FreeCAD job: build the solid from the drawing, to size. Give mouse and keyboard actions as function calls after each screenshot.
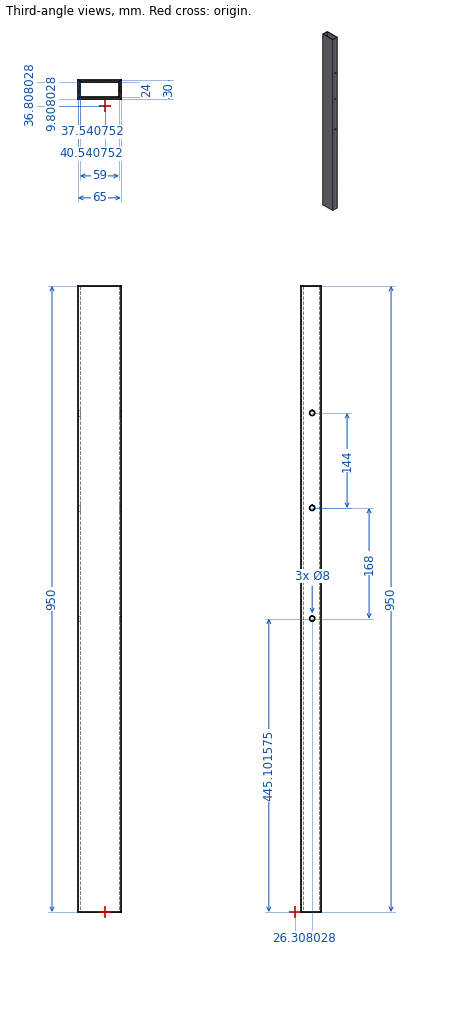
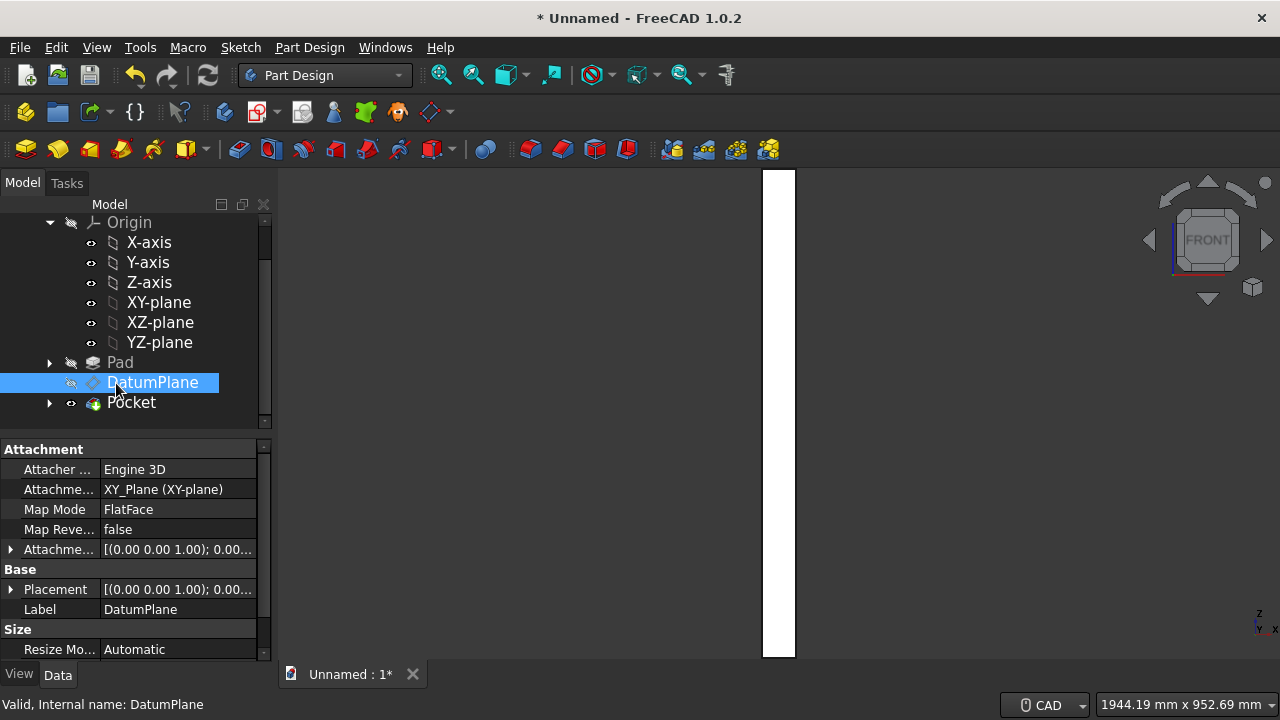
key(6)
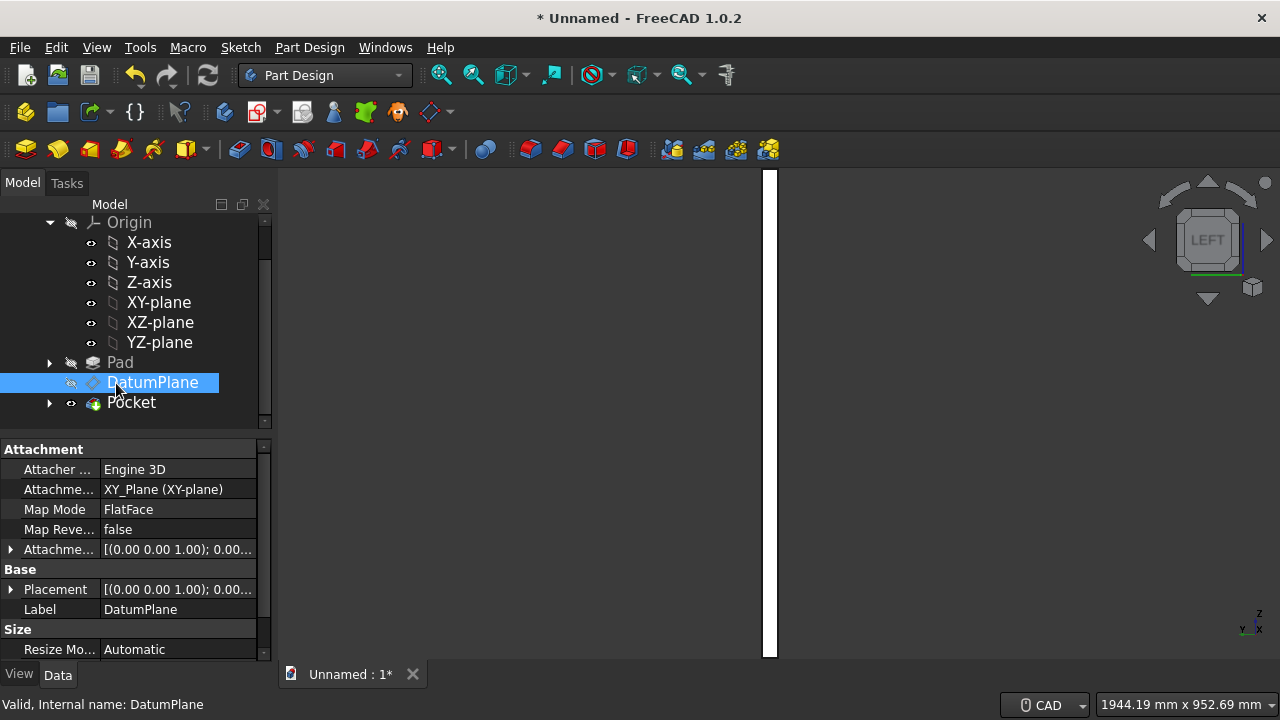
key(2)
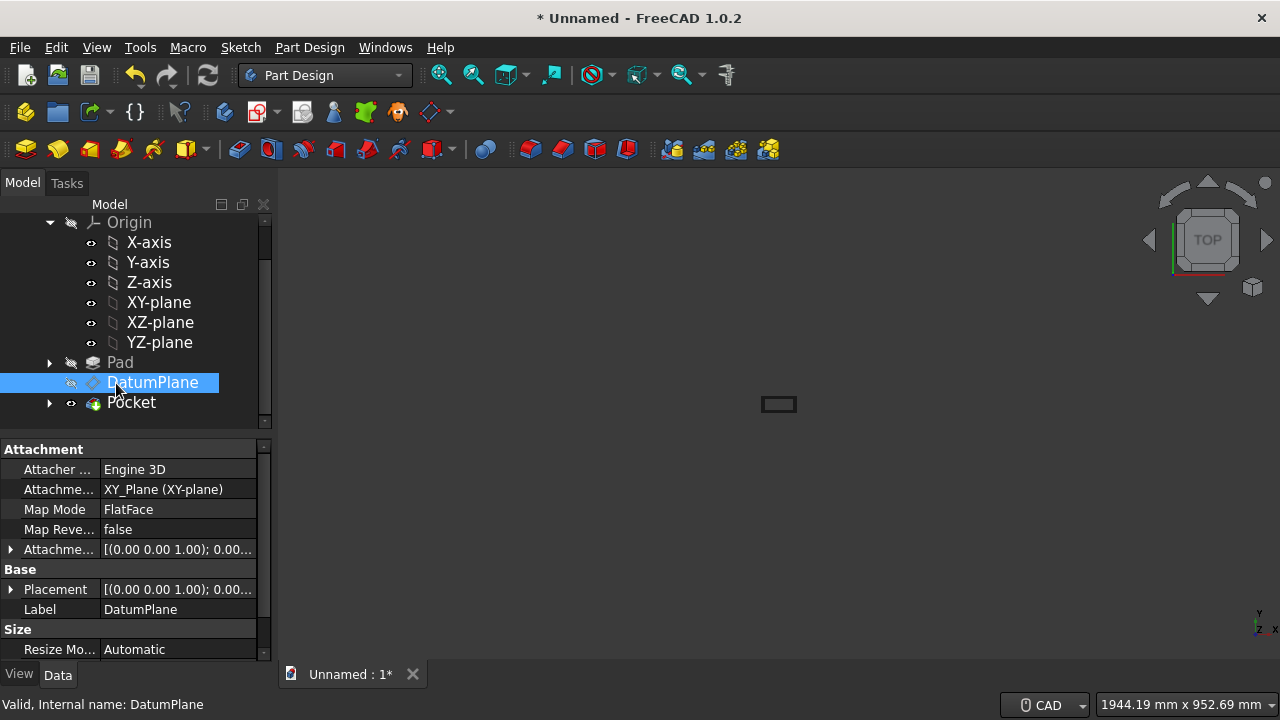
click(442, 76)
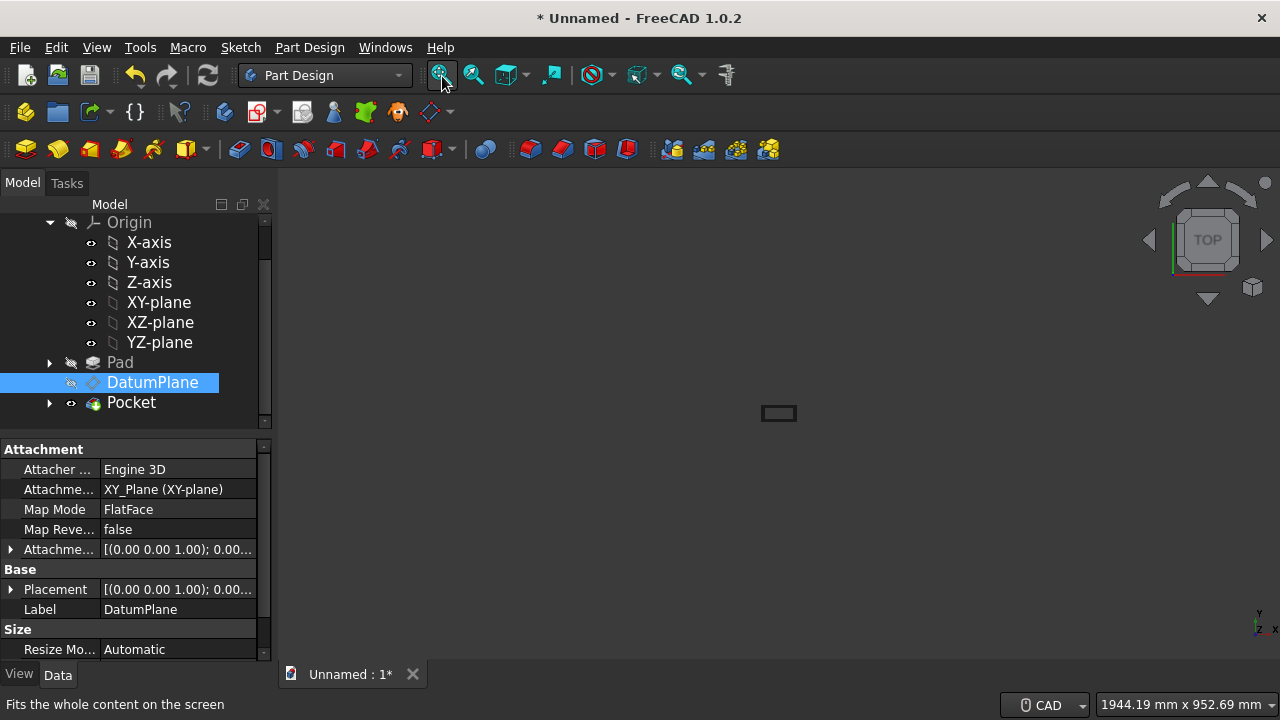
key(1)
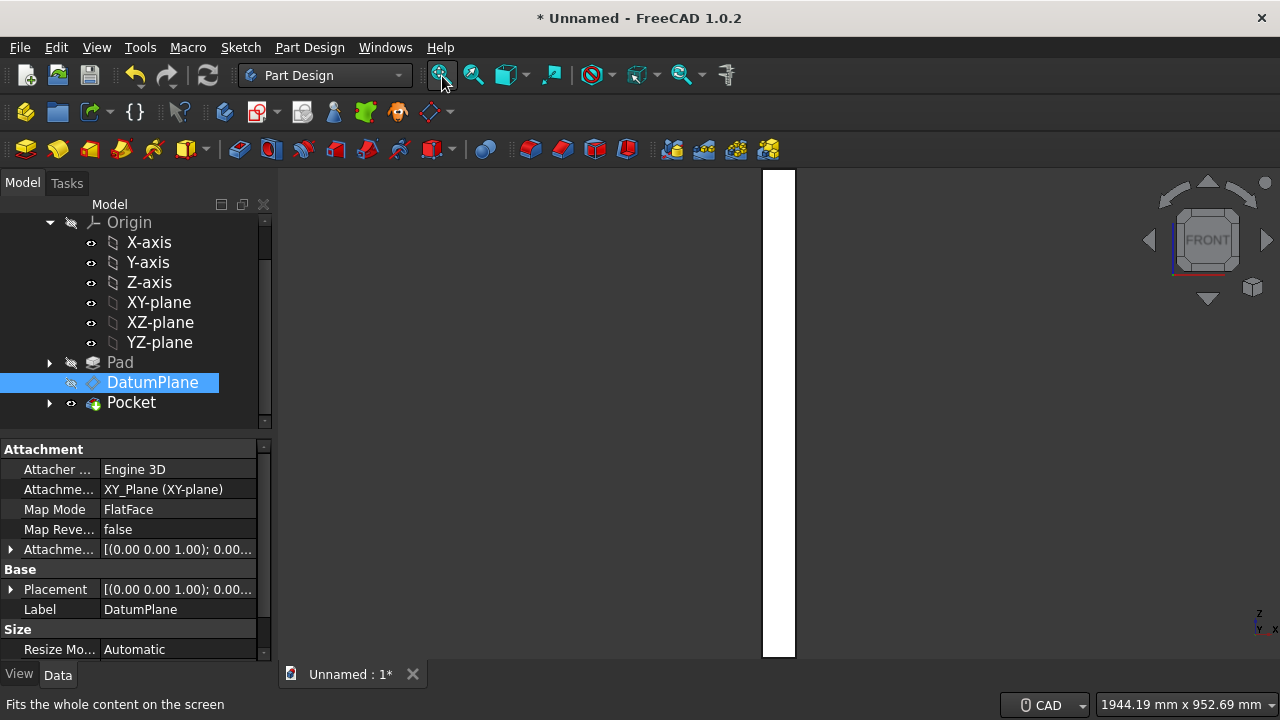
click(136, 343)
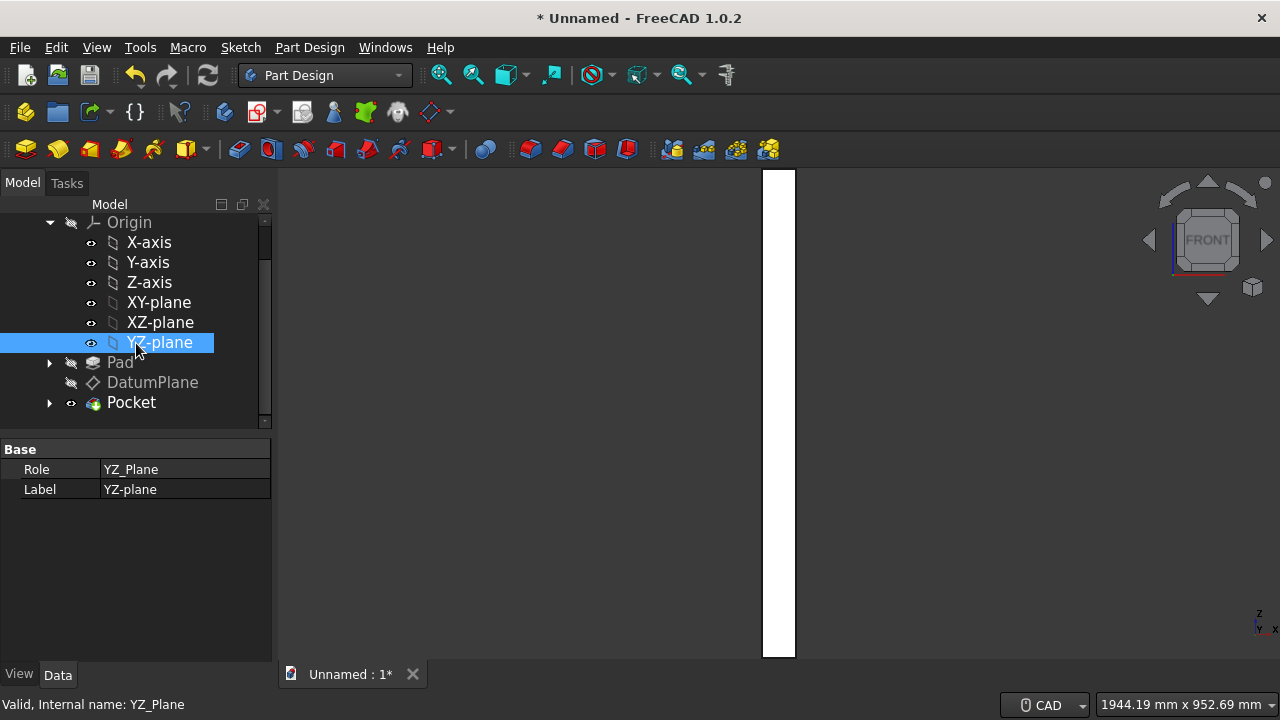
click(430, 112)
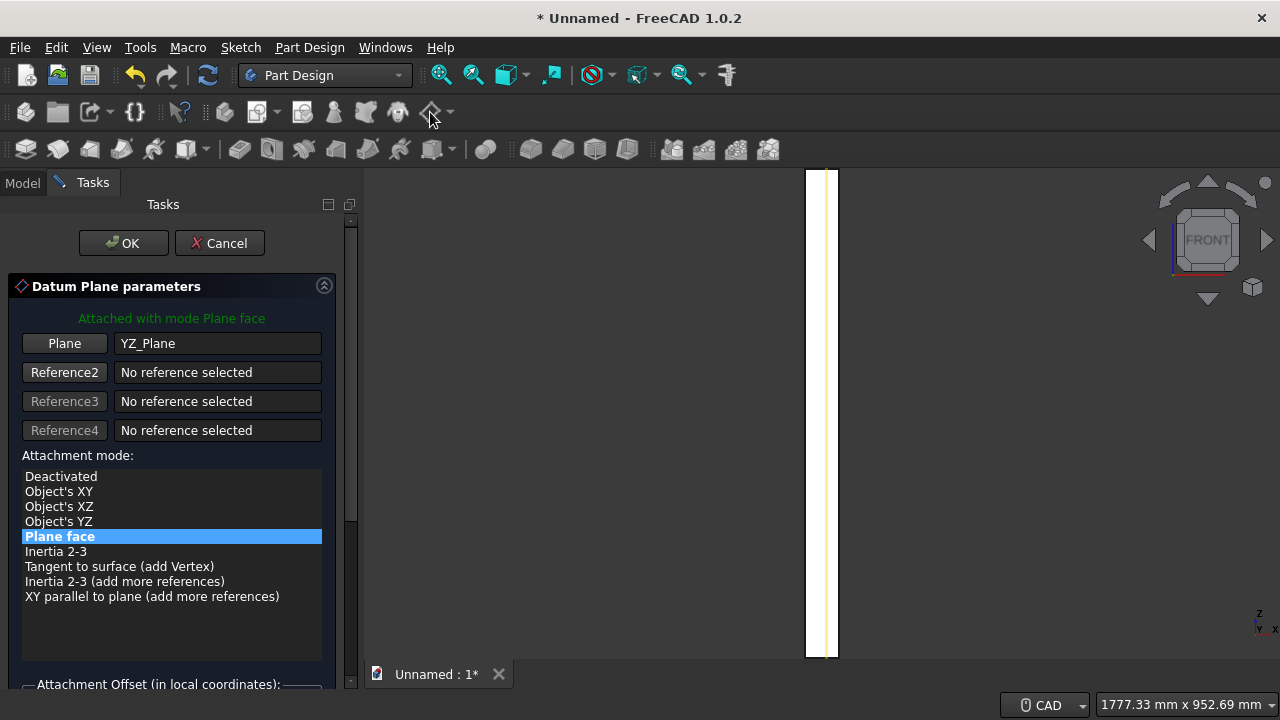
scroll(351, 451, down, 3)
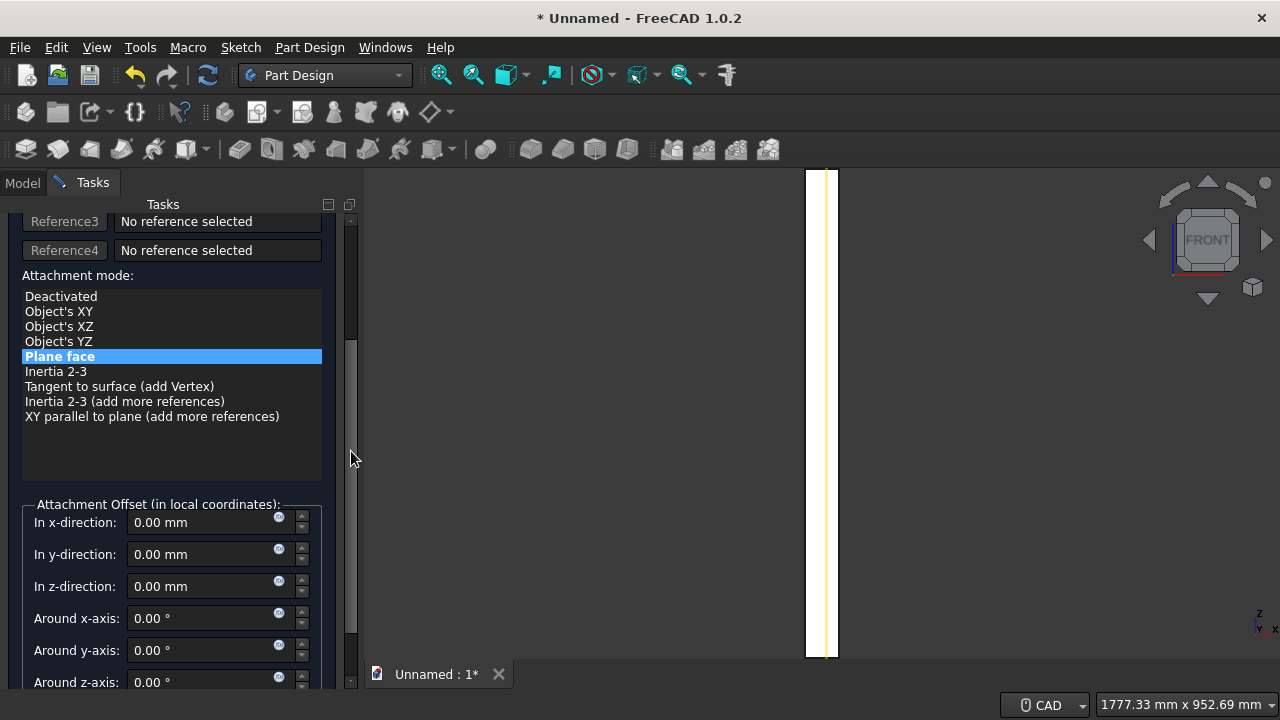
triple_click(210, 586)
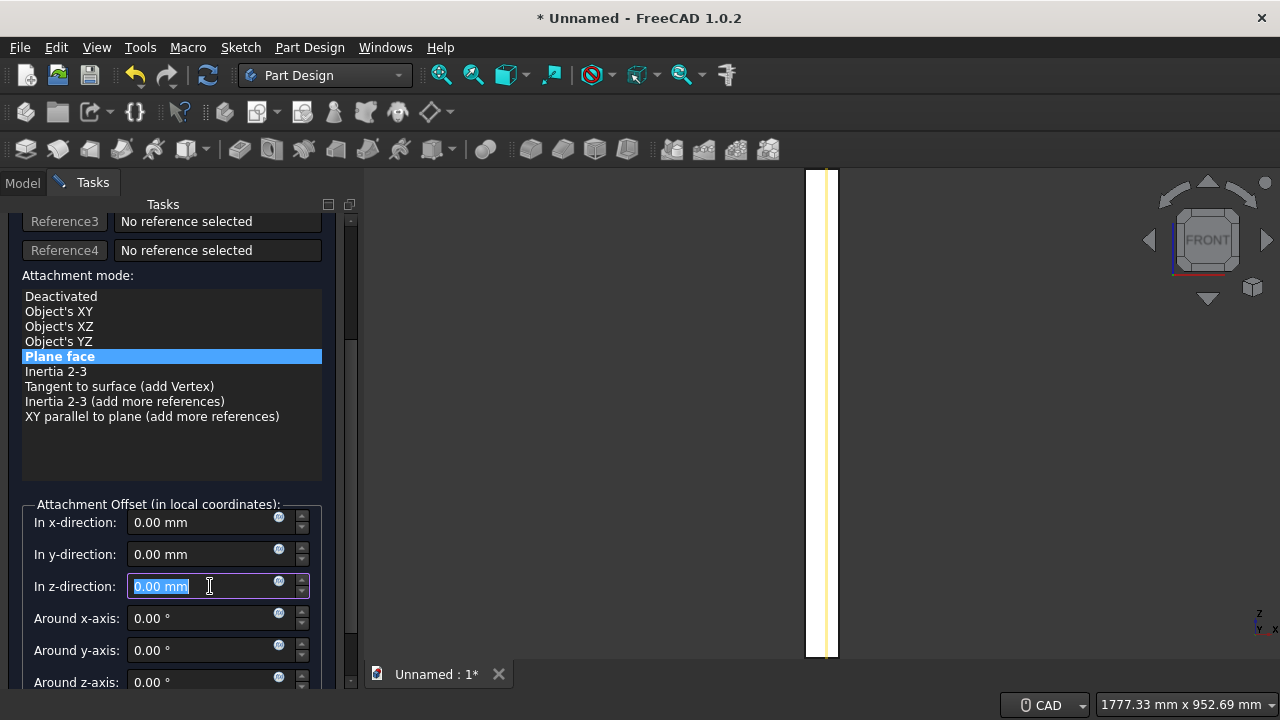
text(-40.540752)
key(Tab)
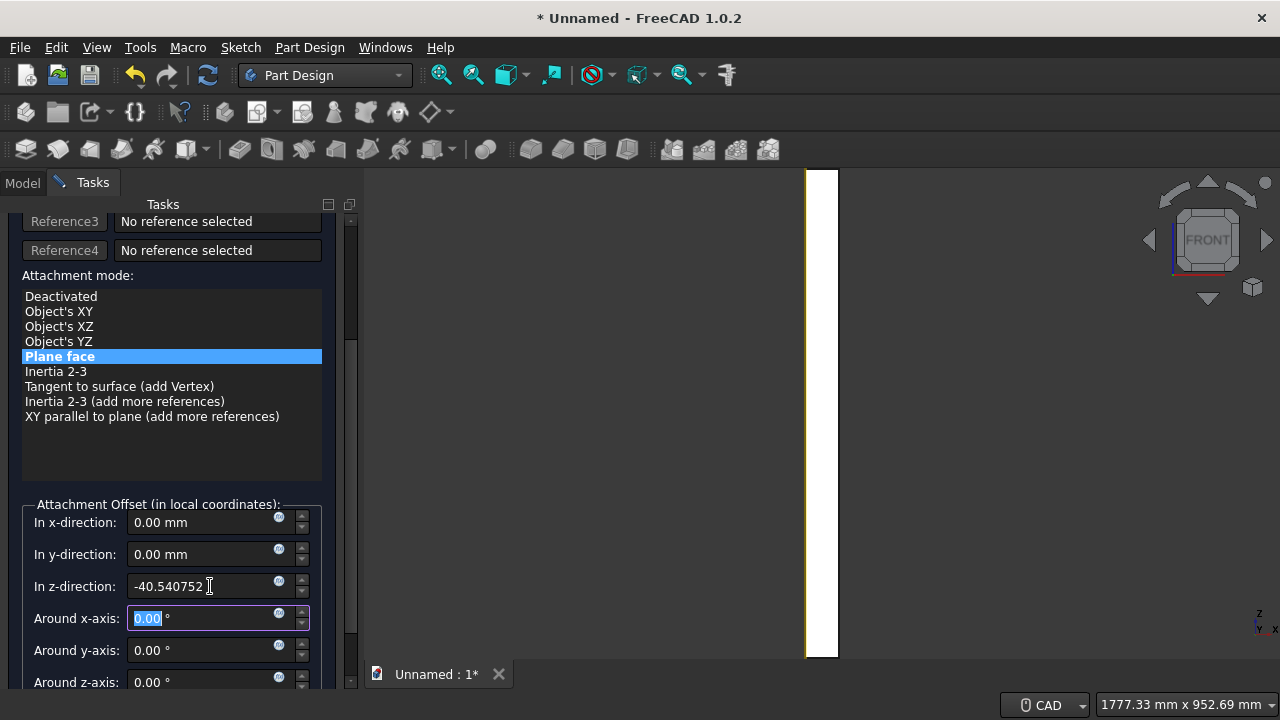
scroll(351, 451, up, 4)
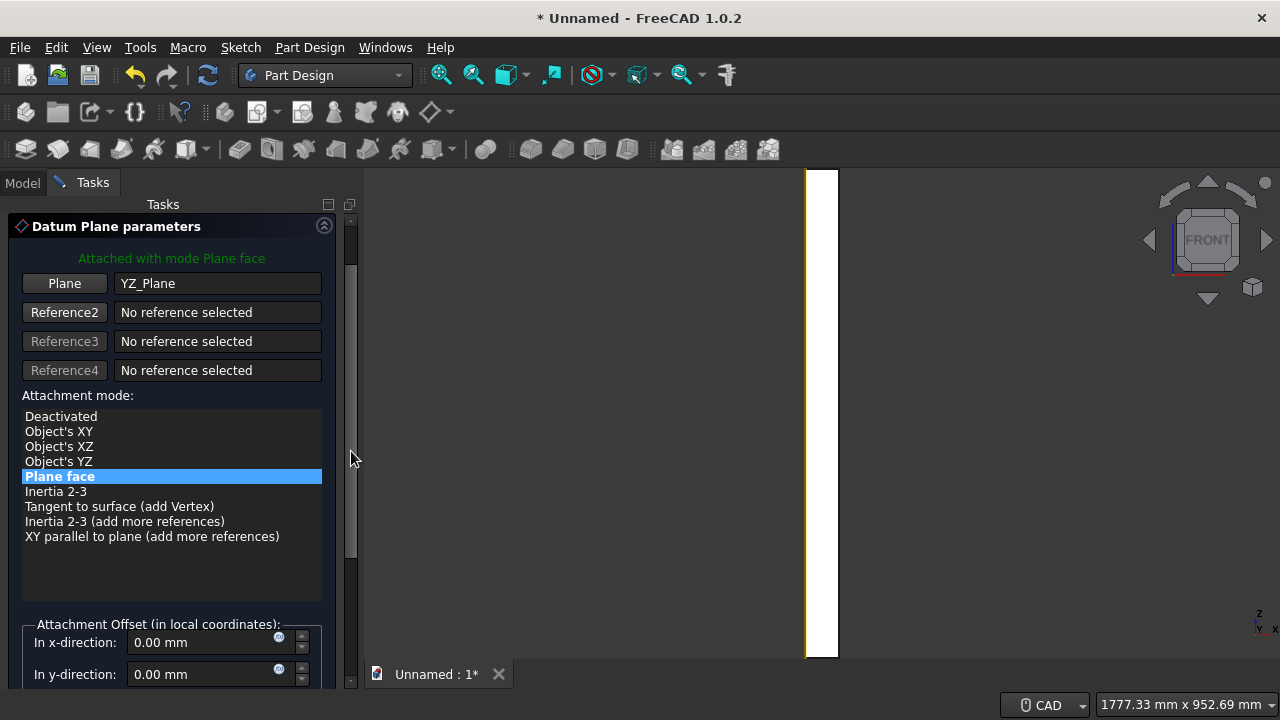
click(124, 243)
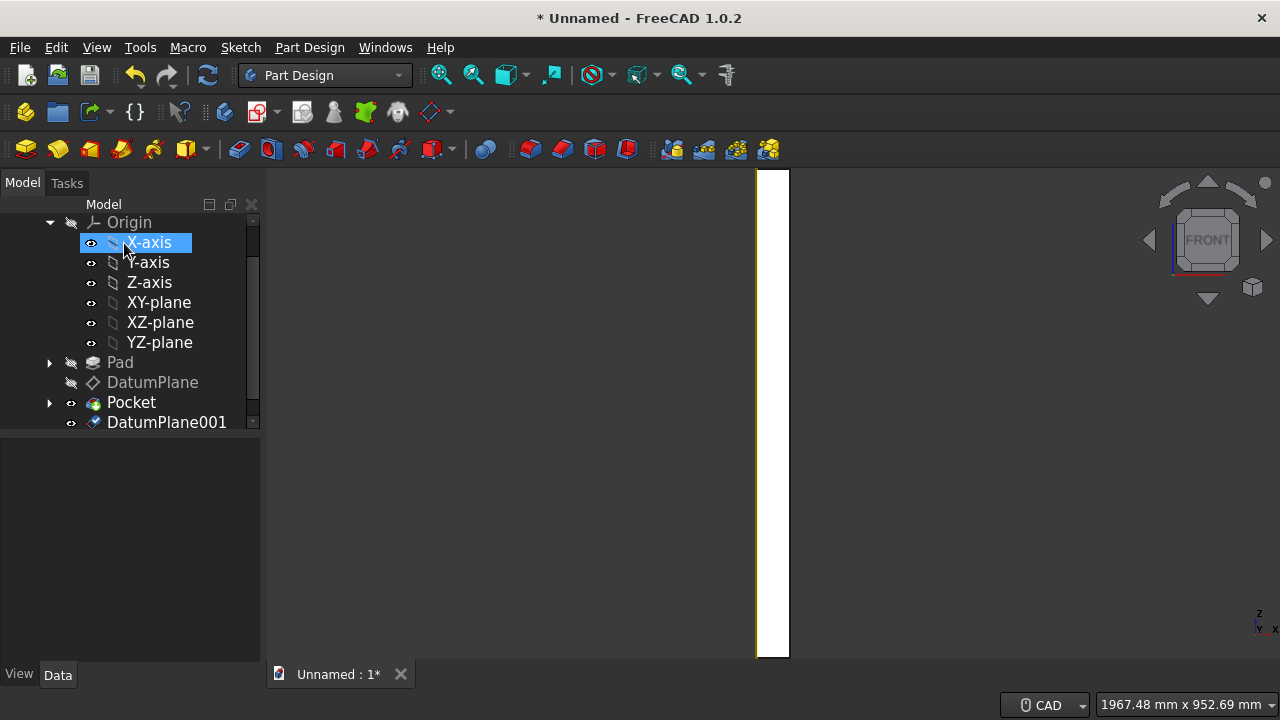
click(116, 423)